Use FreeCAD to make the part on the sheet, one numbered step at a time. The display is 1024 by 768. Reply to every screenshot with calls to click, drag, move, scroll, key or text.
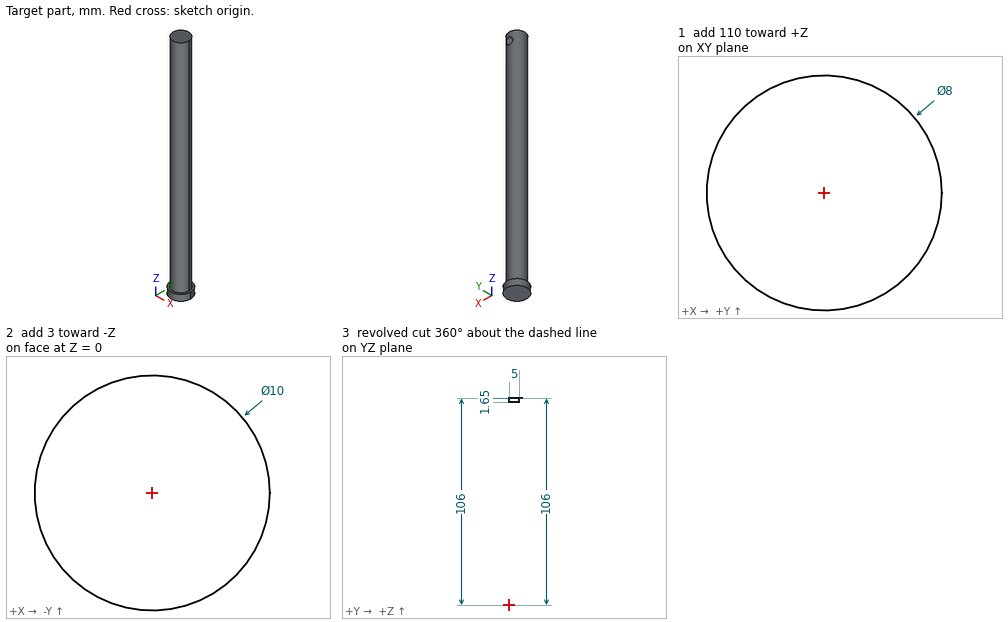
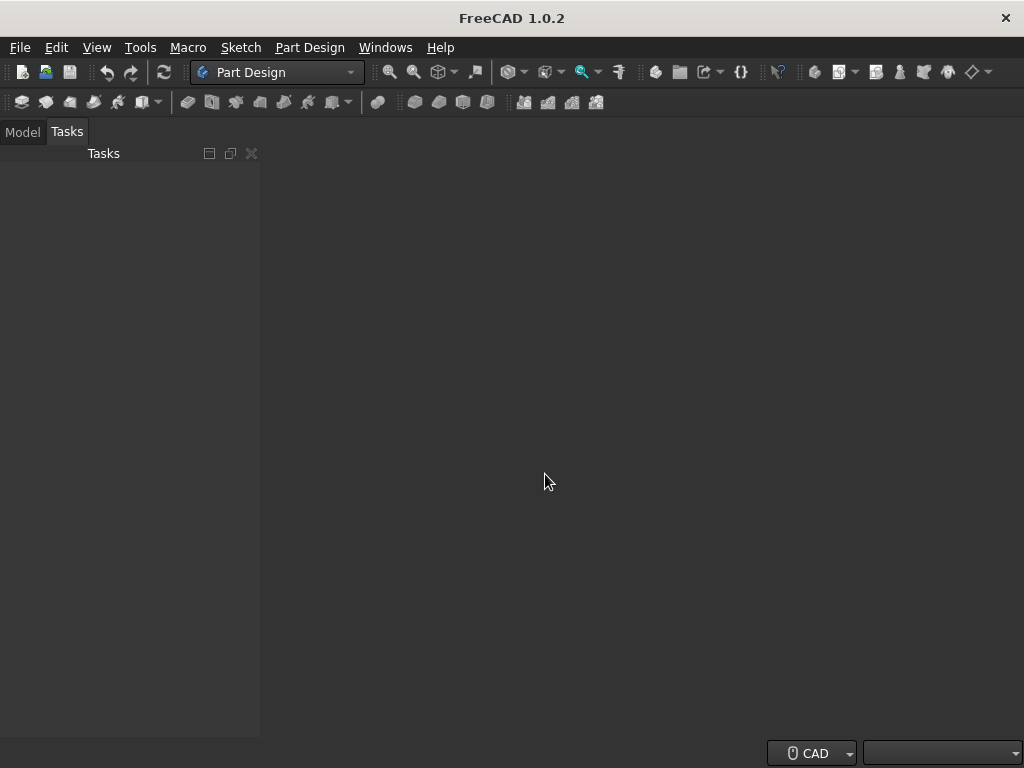
click(22, 72)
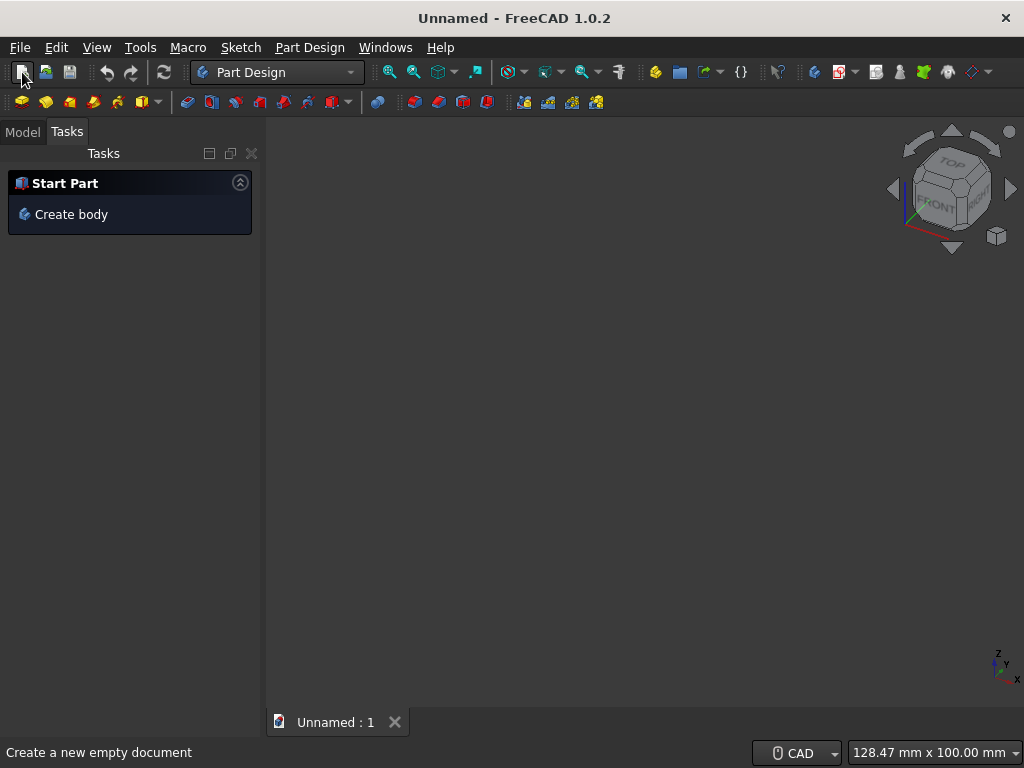
click(840, 72)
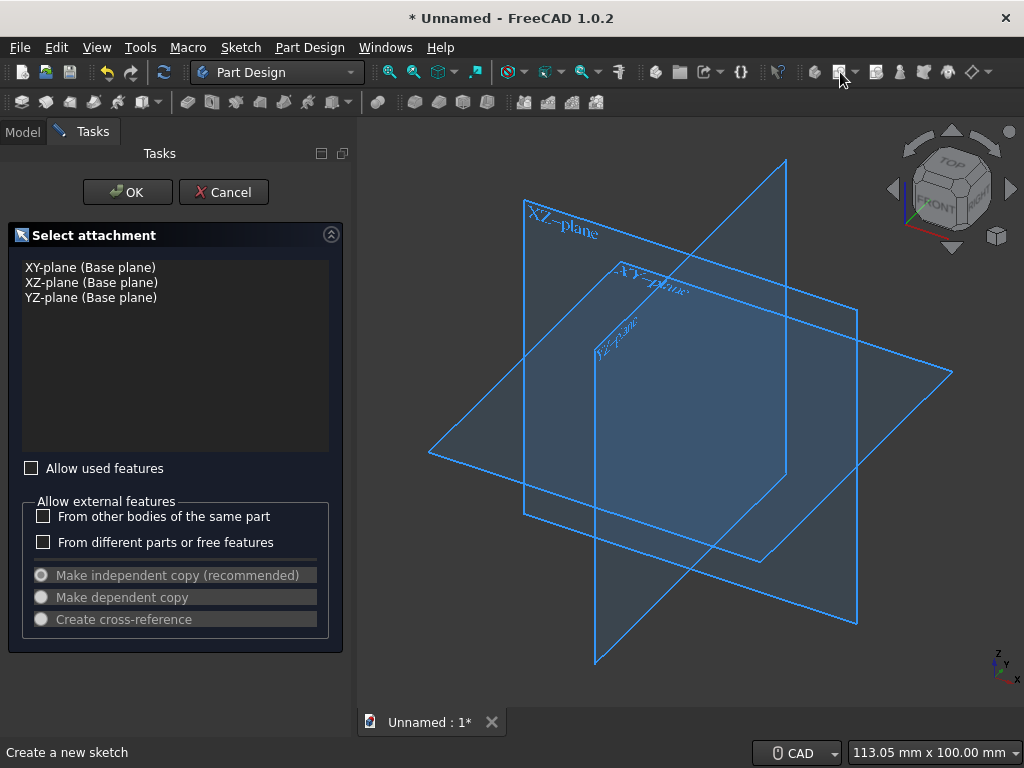
click(82, 268)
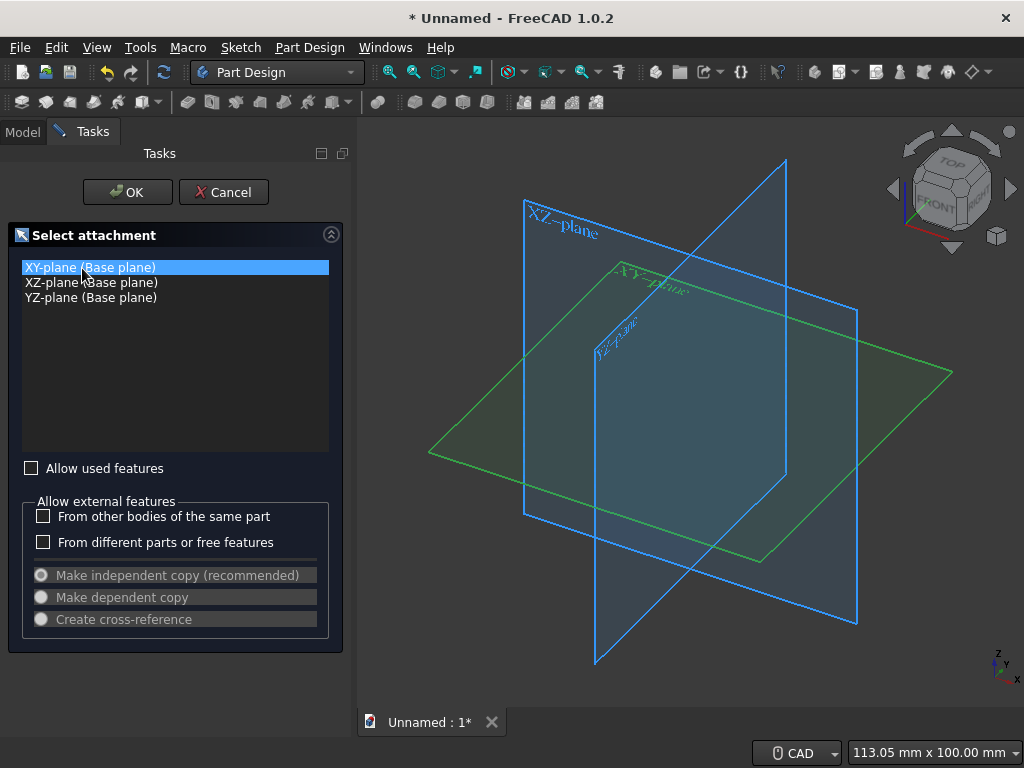
click(128, 192)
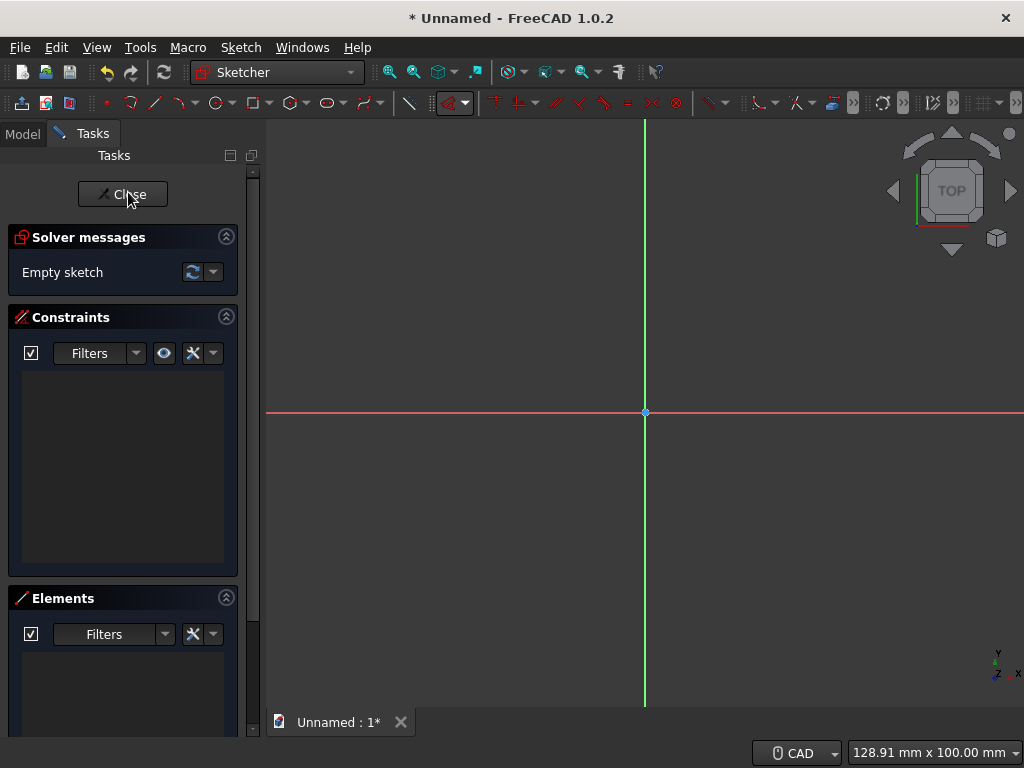
scroll(656, 413, up, 10)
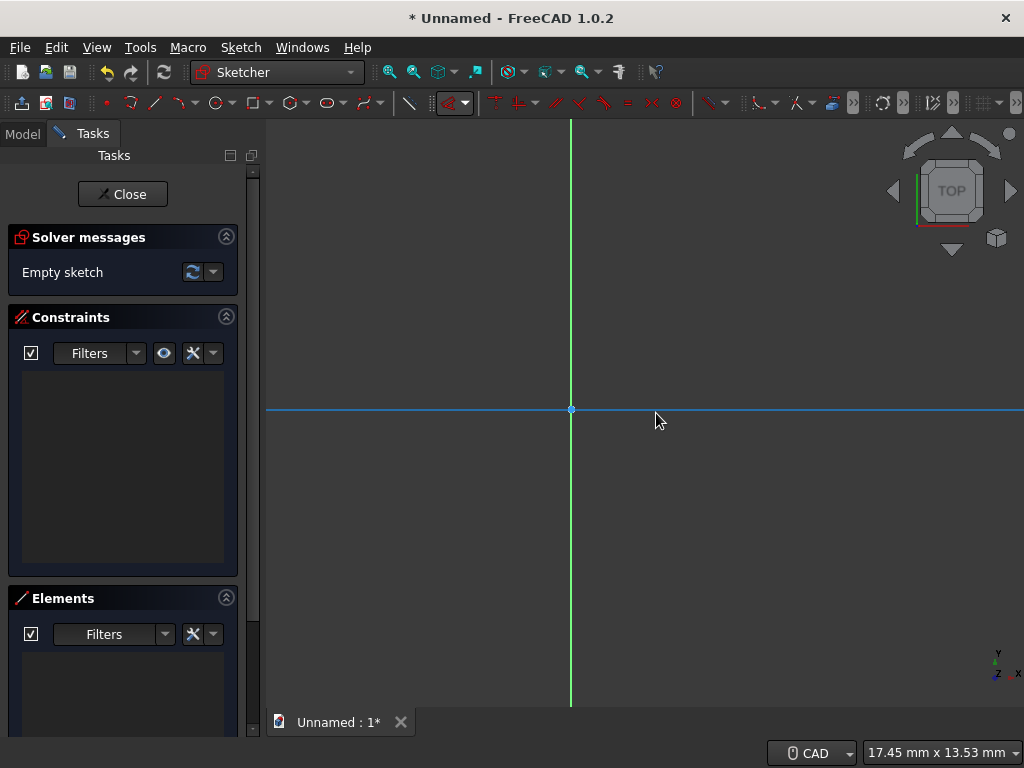
click(216, 104)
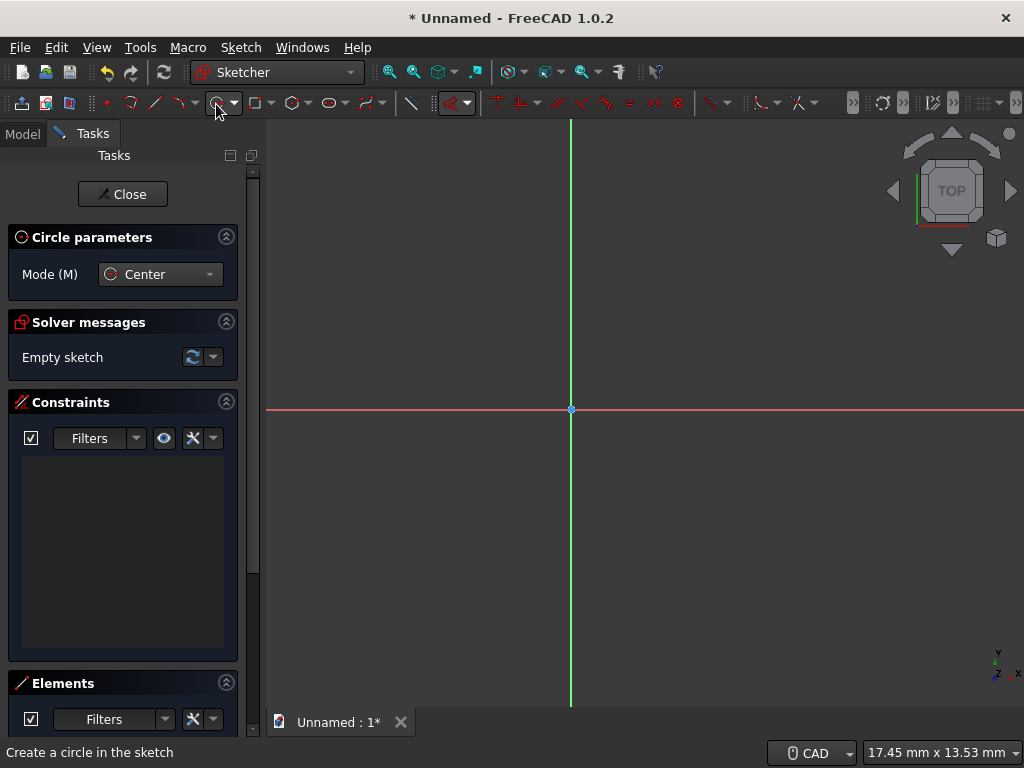
click(571, 410)
click(694, 287)
key(Escape)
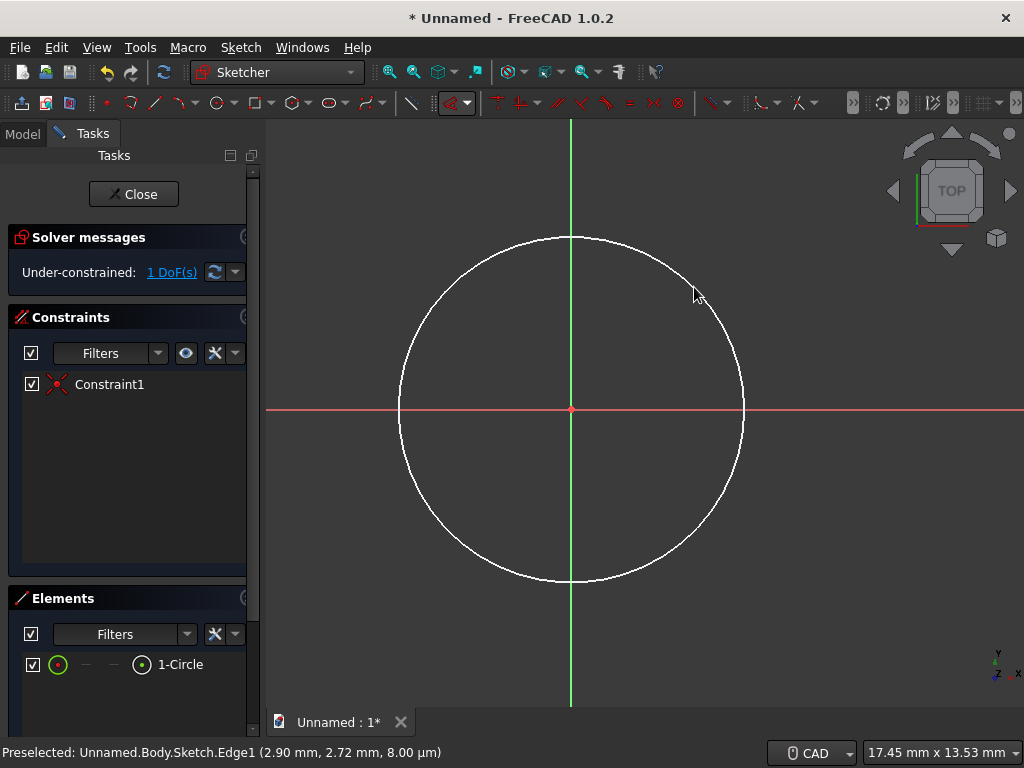
click(450, 104)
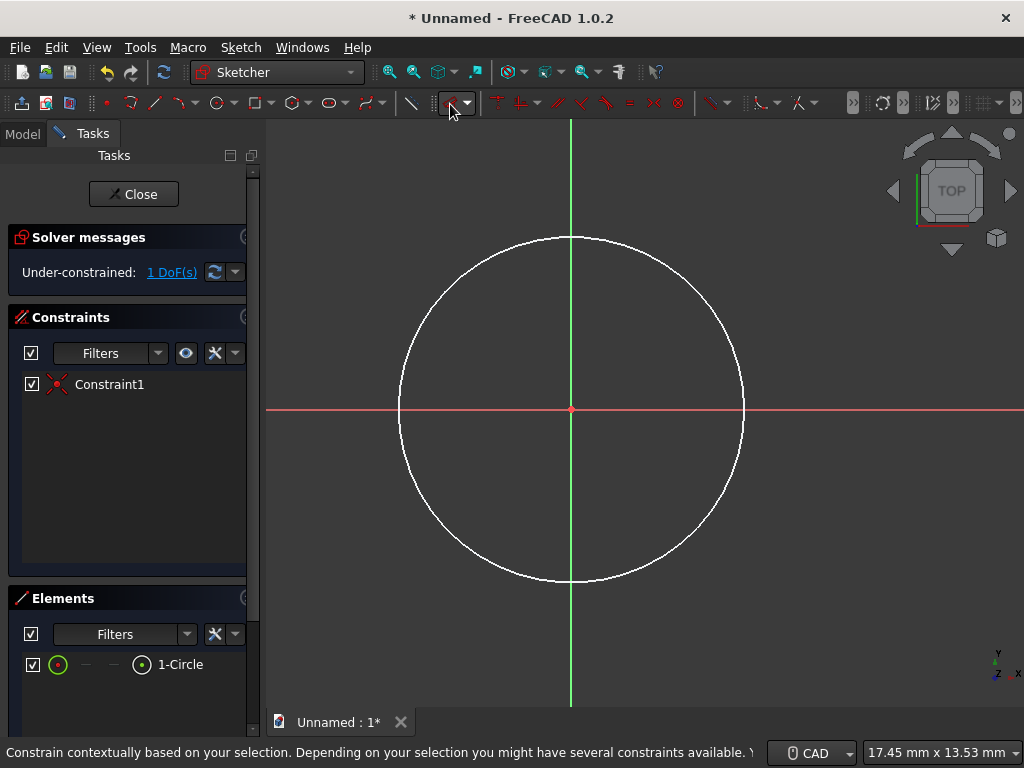
click(693, 287)
click(716, 264)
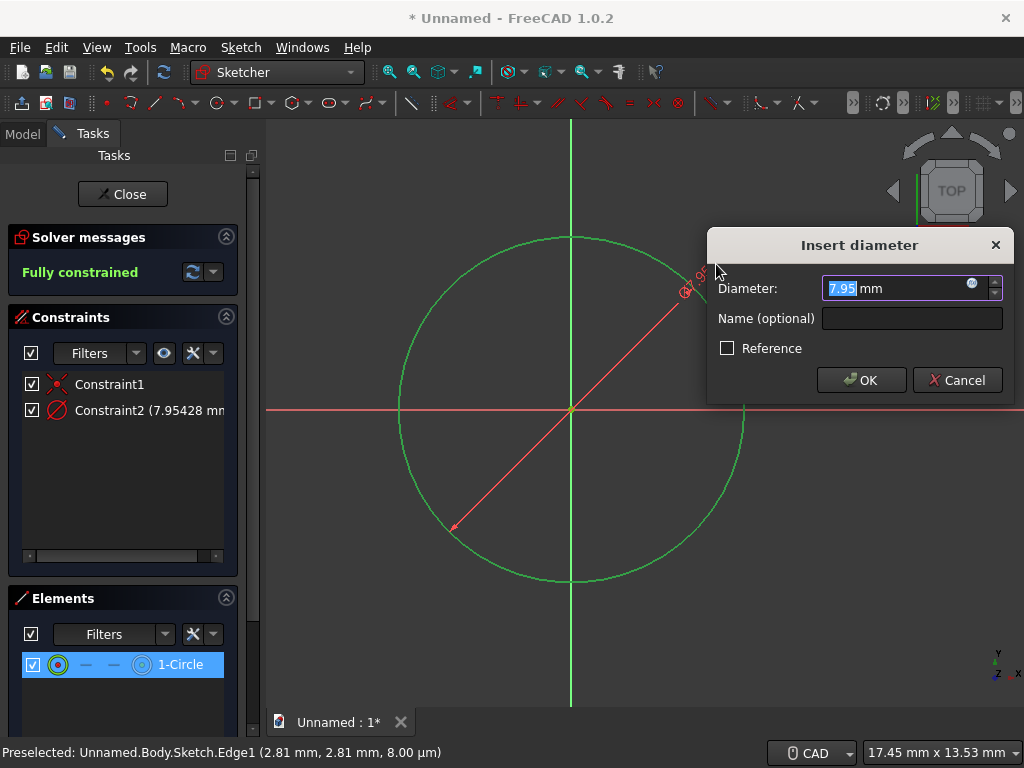
text(8)
key(Return)
key(Escape)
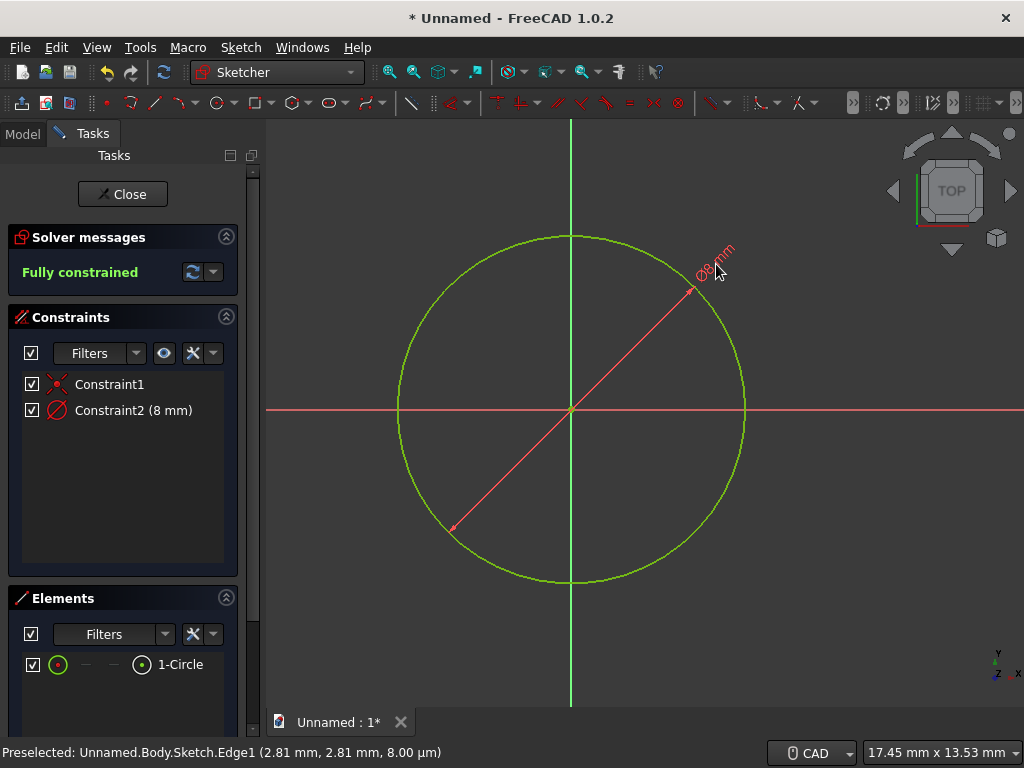
click(123, 194)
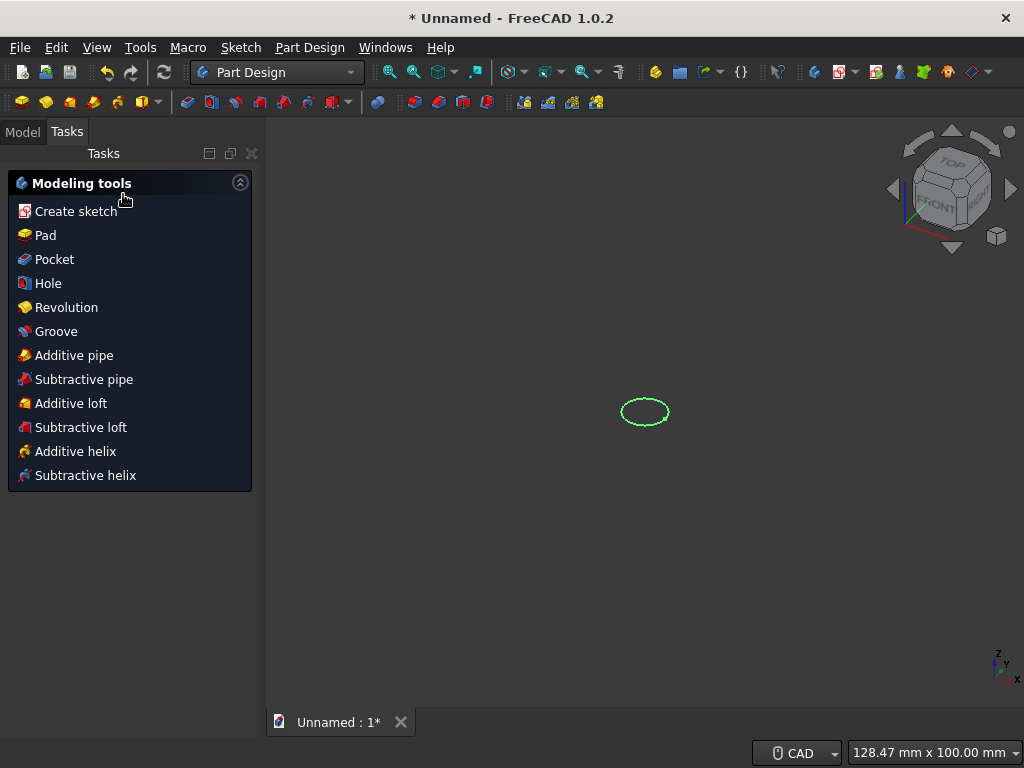
click(22, 102)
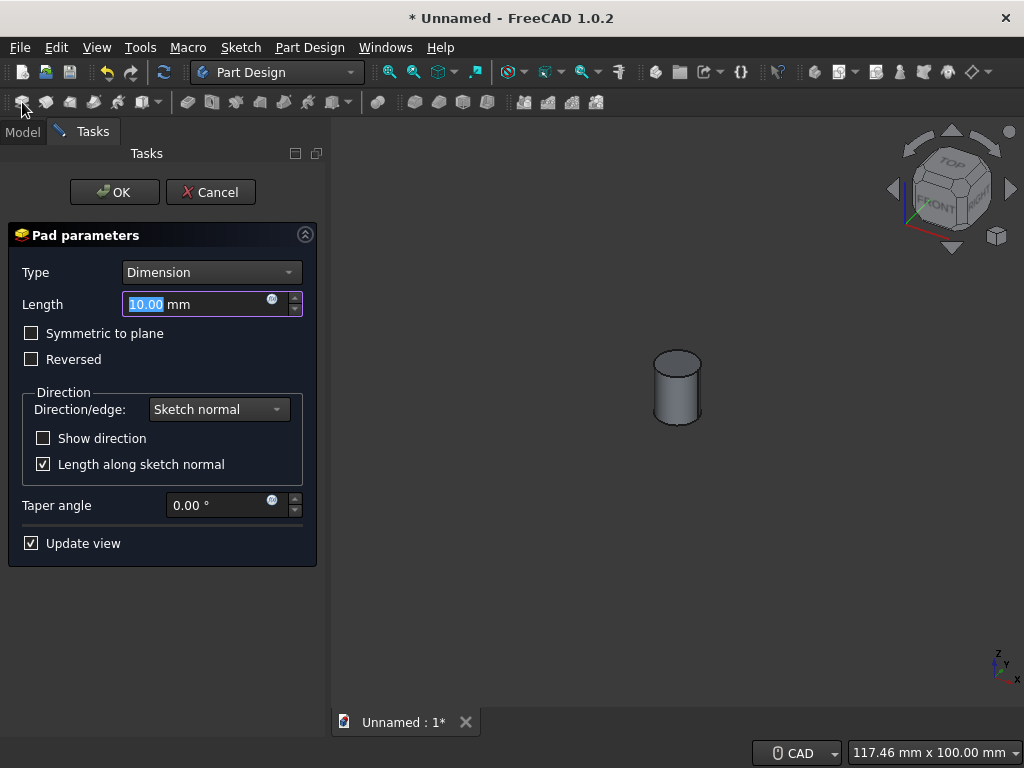
text(110)
key(Tab)